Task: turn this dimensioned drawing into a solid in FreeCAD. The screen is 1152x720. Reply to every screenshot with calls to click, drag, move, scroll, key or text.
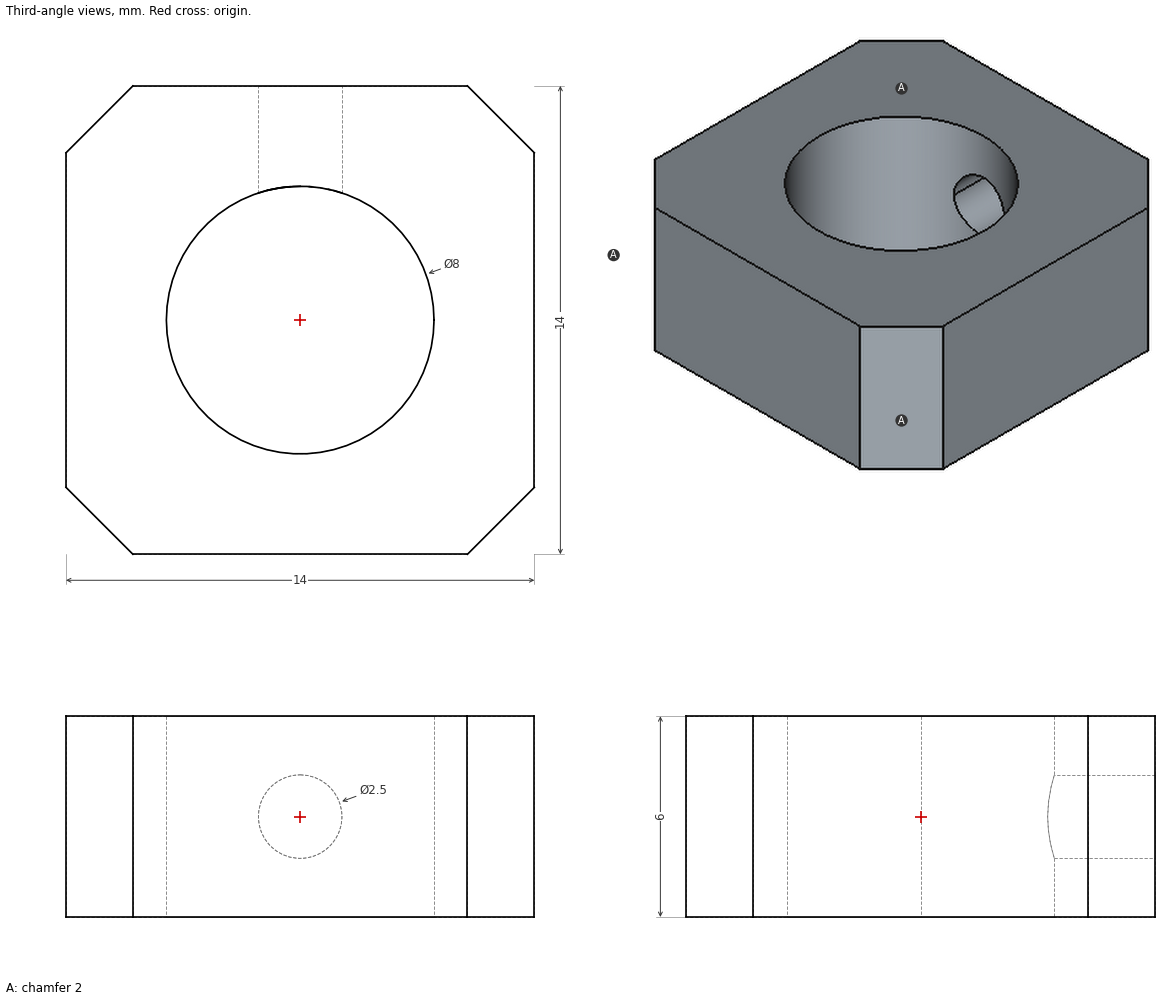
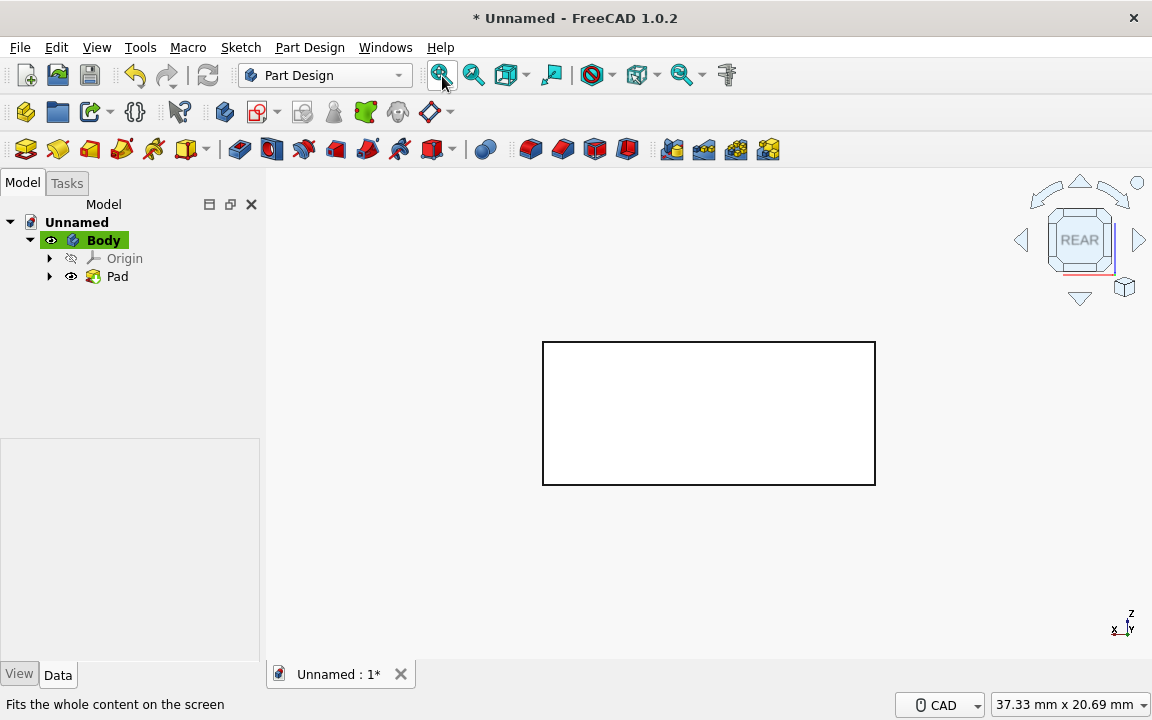
click(442, 76)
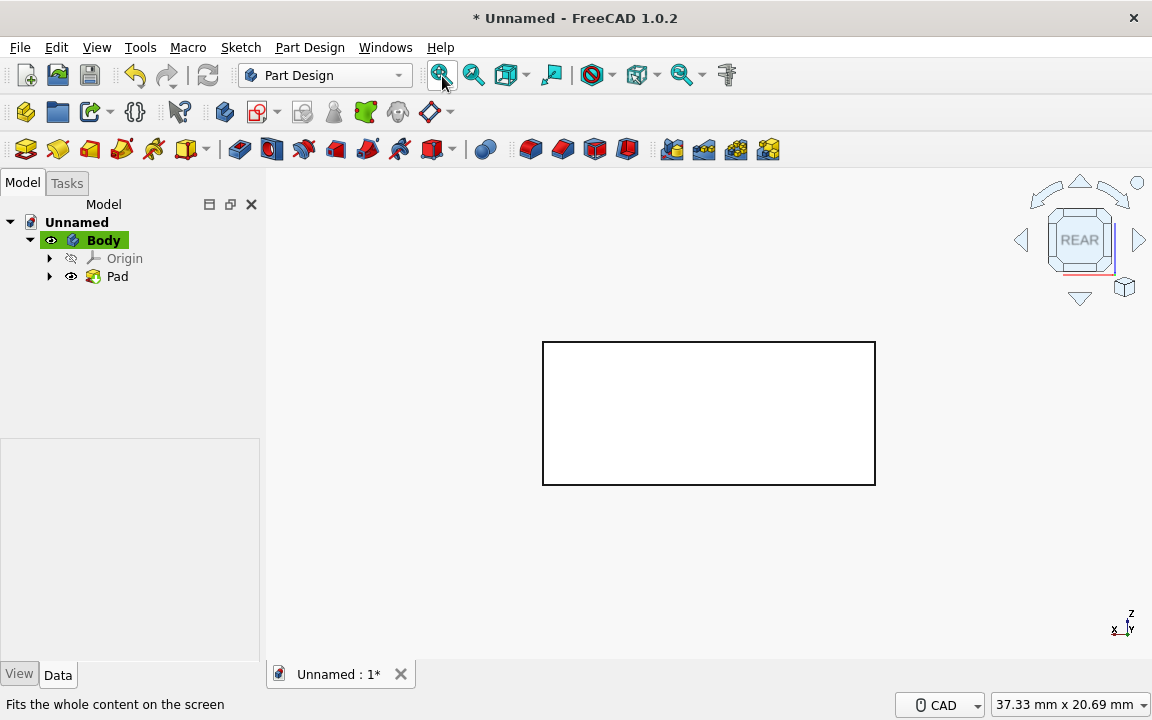
click(614, 413)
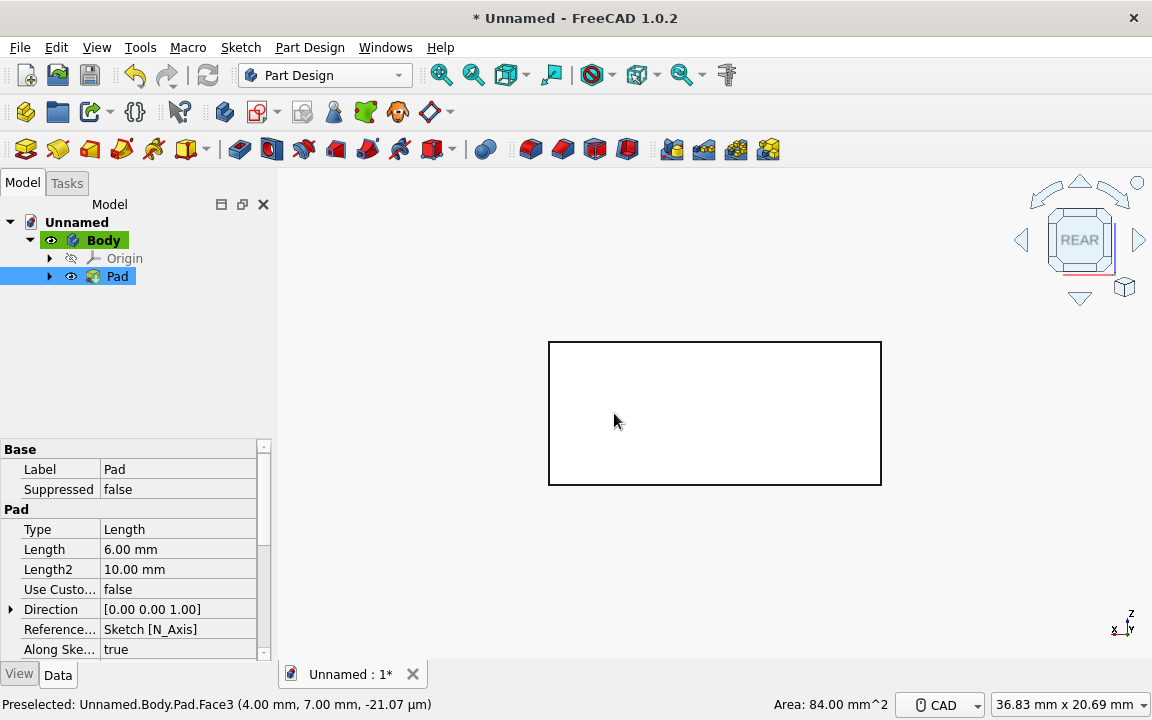
click(258, 112)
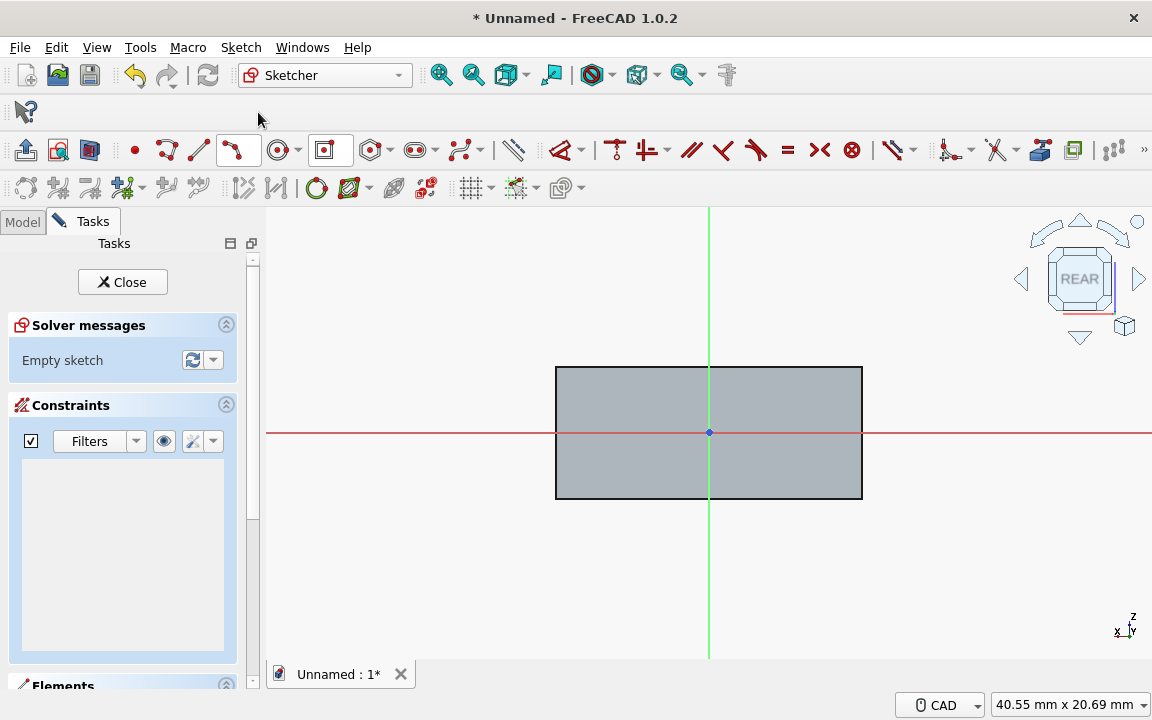
scroll(726, 433, up, 8)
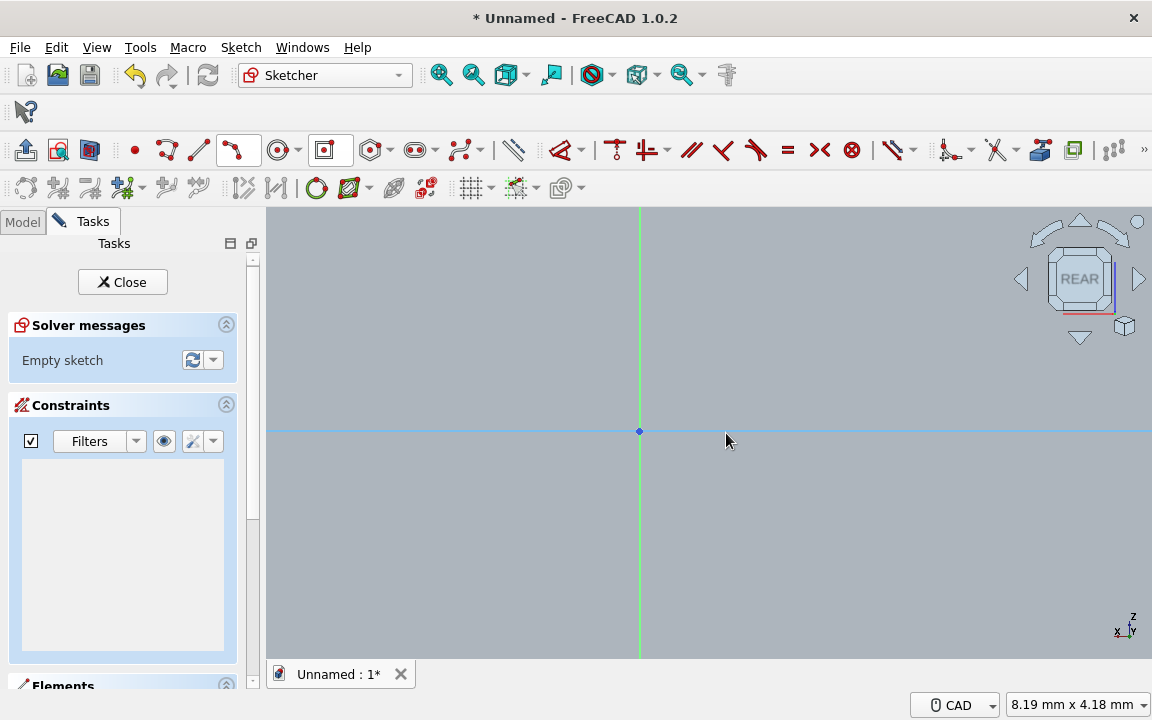
click(278, 150)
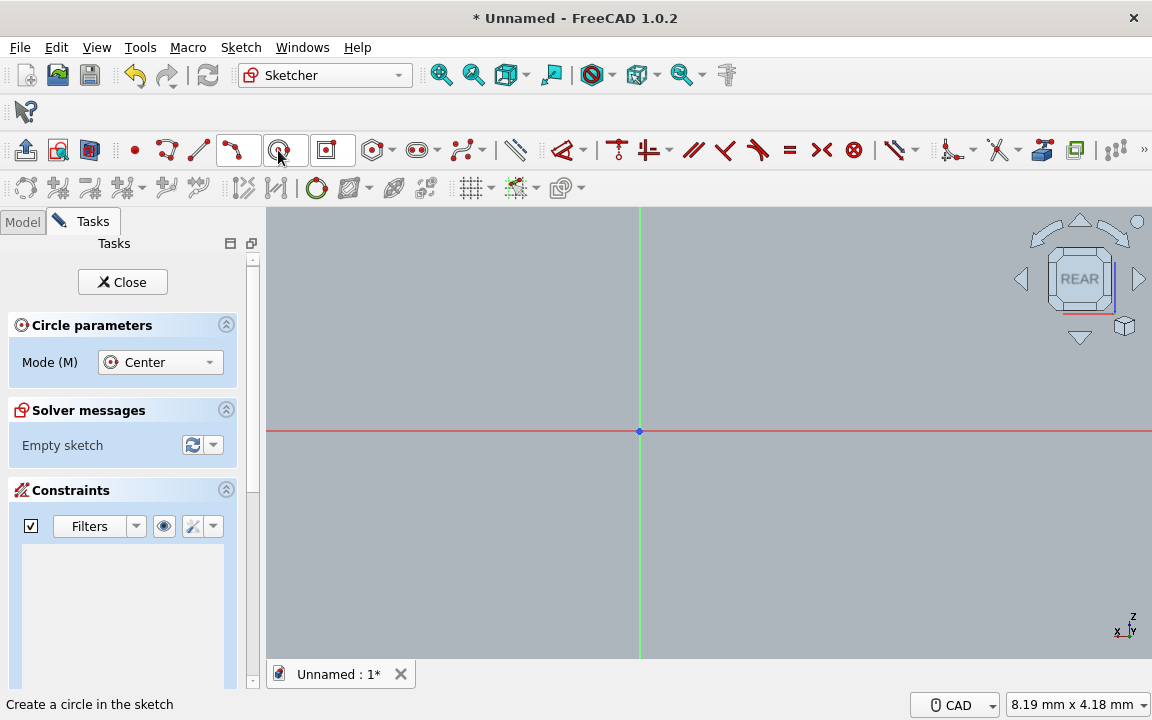
click(640, 431)
click(735, 335)
key(Escape)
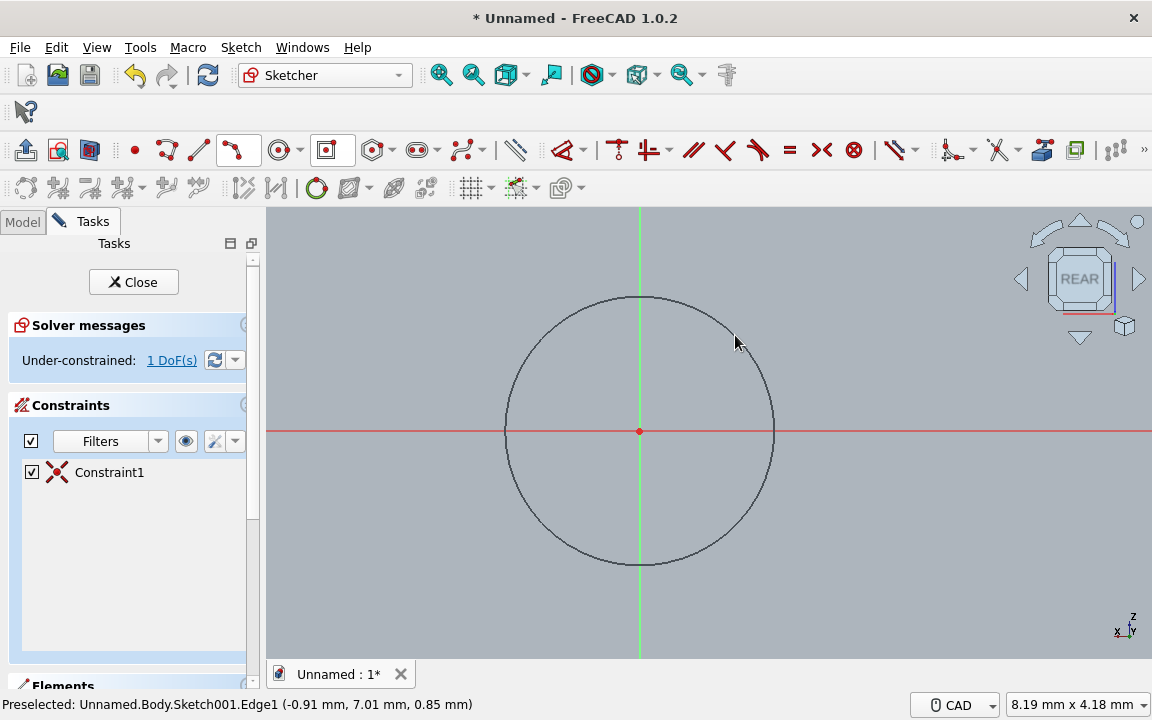
click(562, 150)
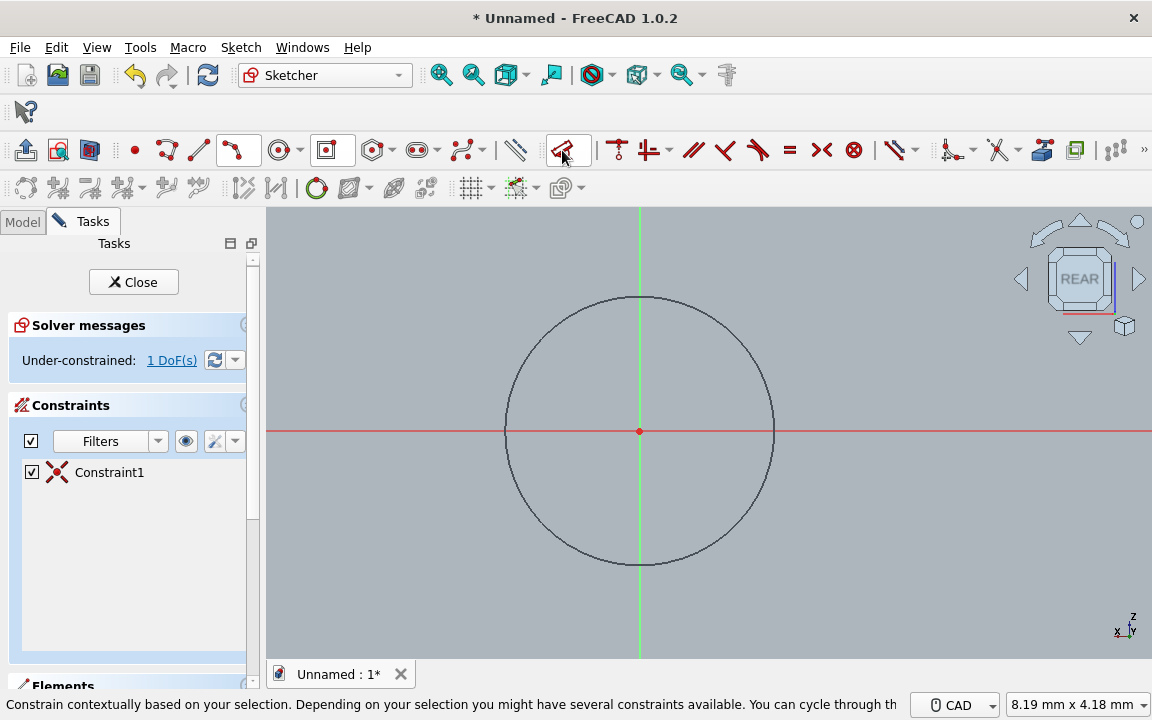
click(735, 336)
click(758, 313)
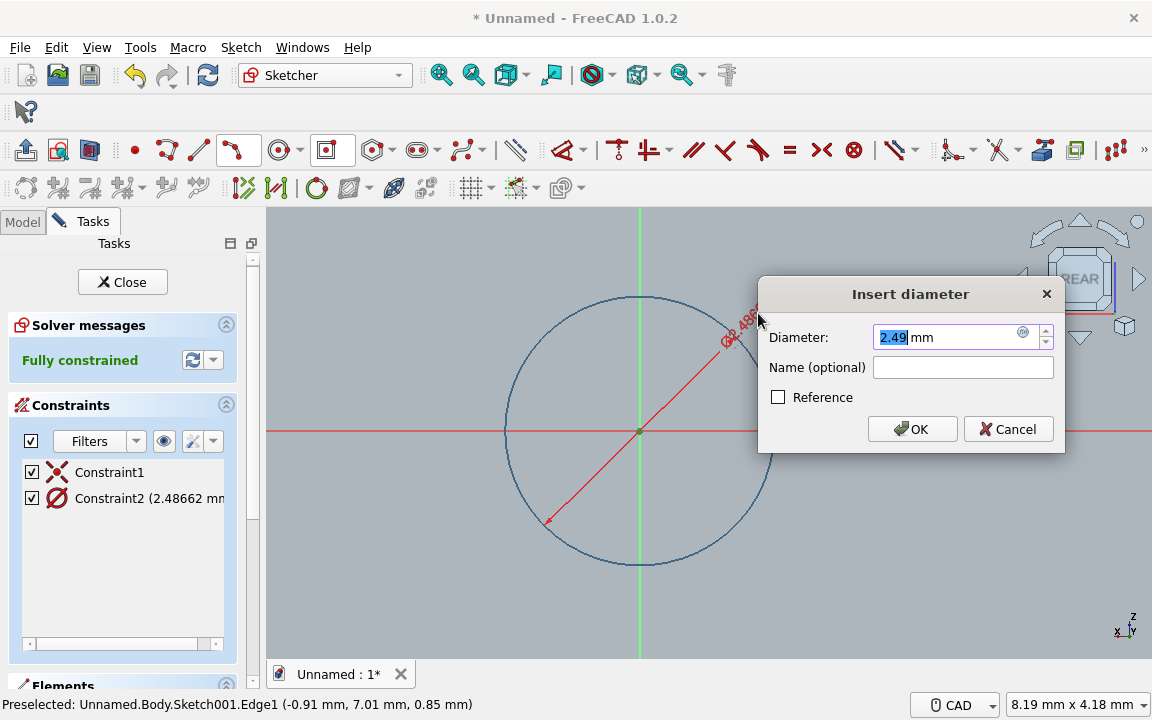
text(2.5)
key(Return)
key(Escape)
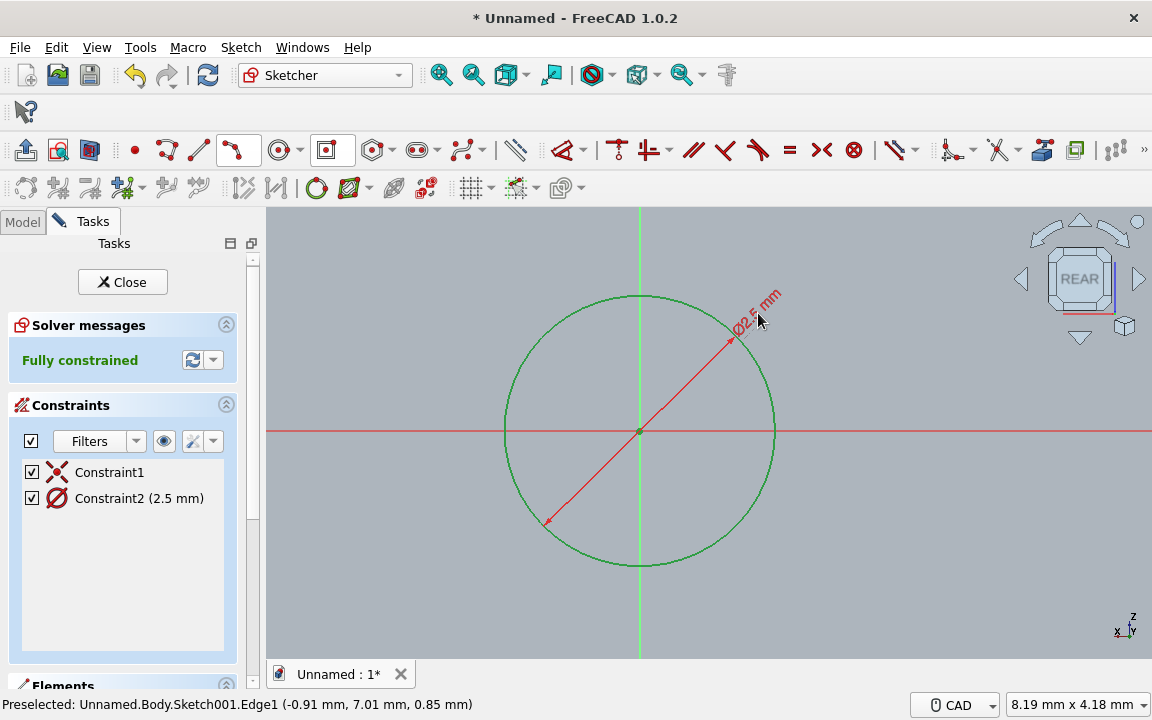
click(123, 282)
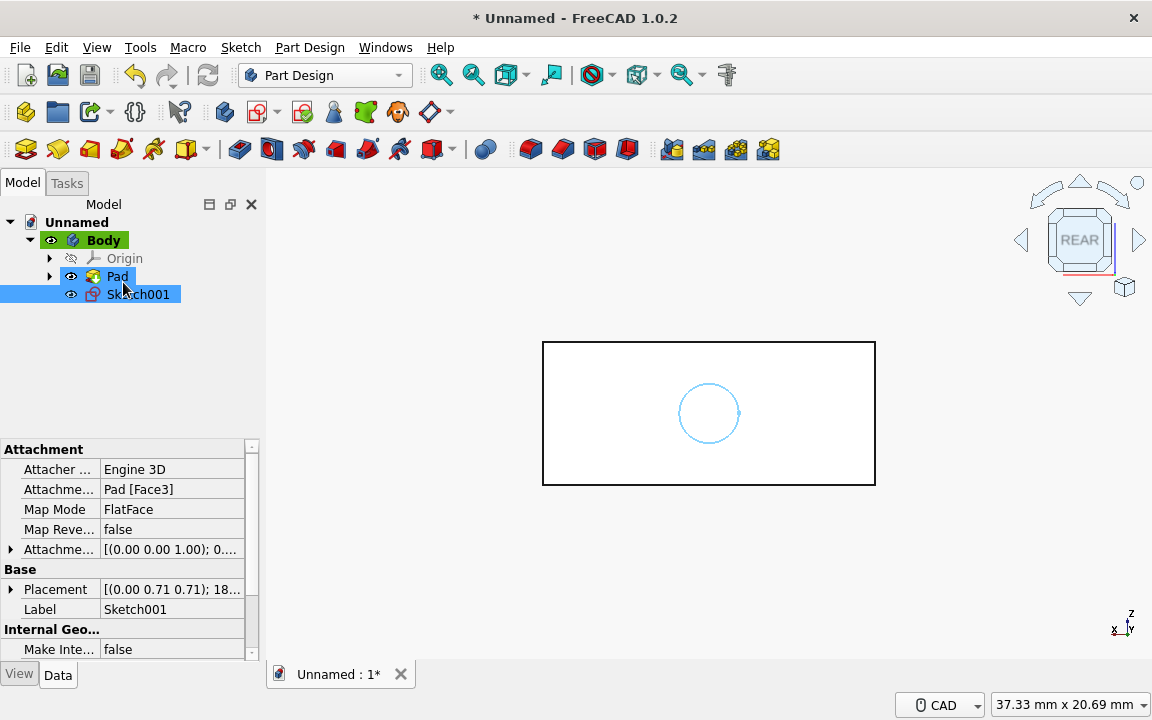
click(240, 150)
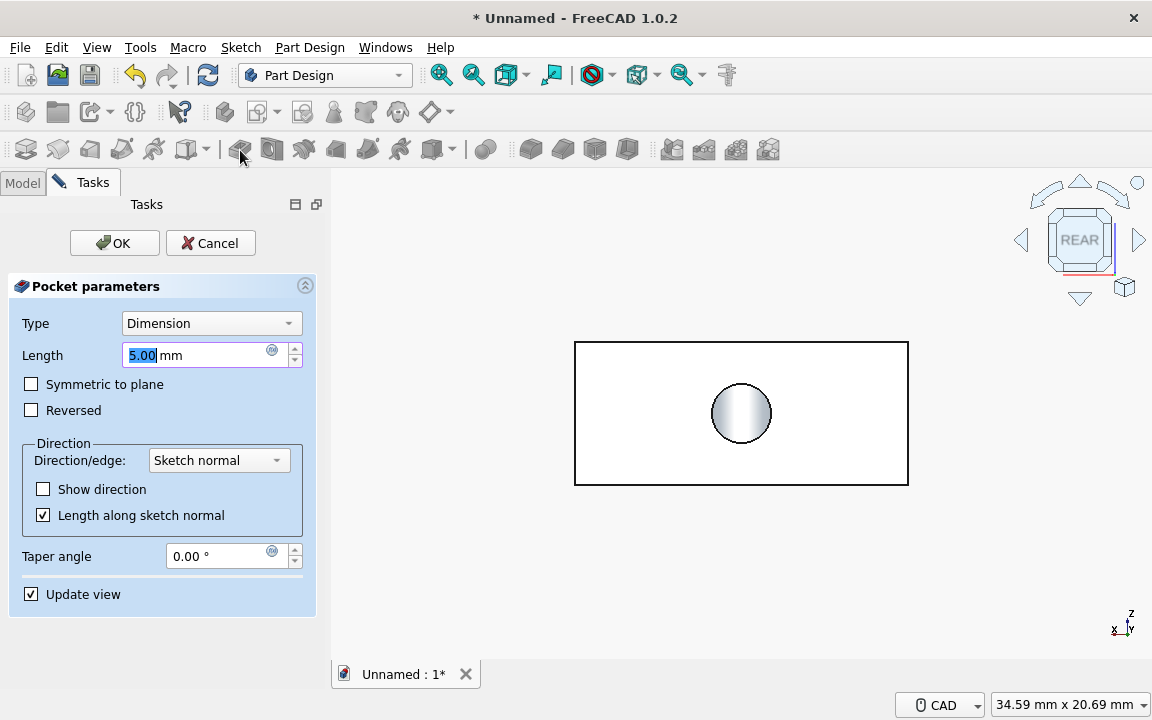
click(212, 324)